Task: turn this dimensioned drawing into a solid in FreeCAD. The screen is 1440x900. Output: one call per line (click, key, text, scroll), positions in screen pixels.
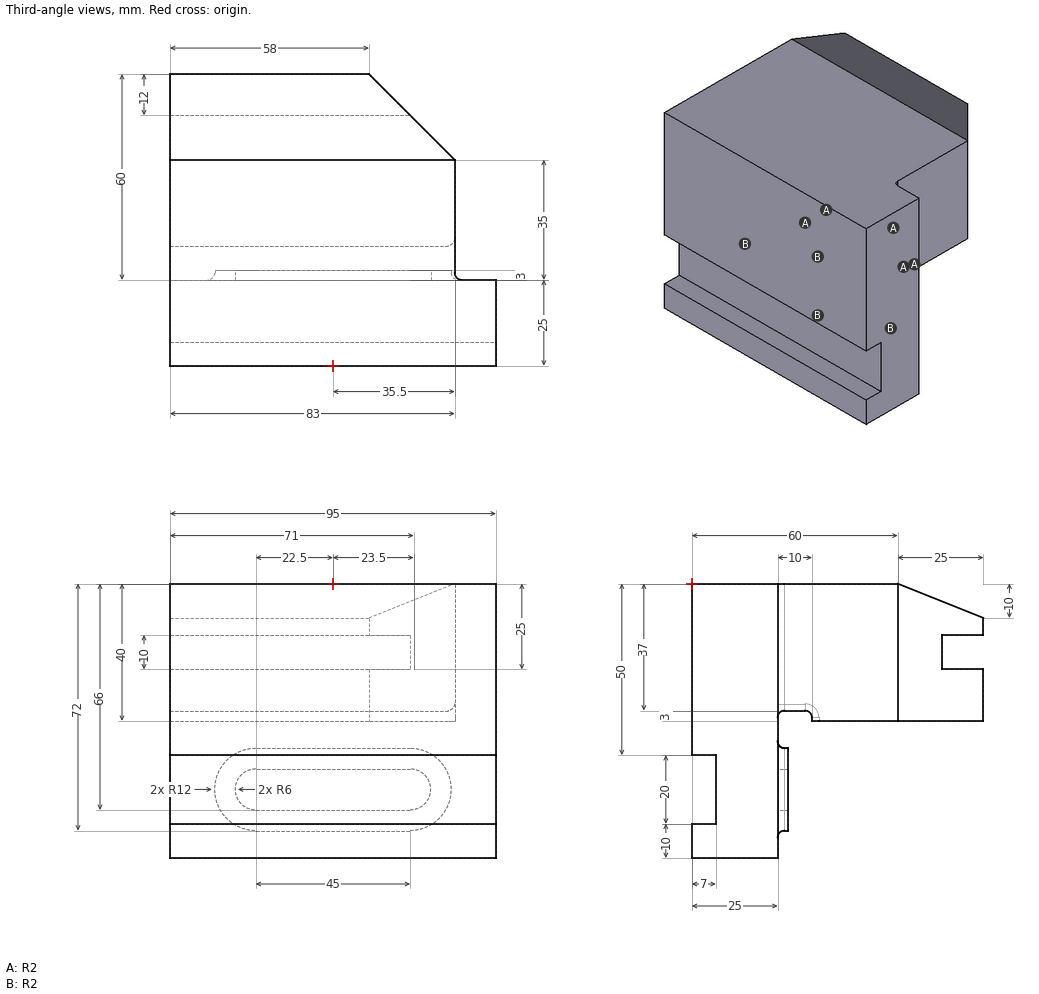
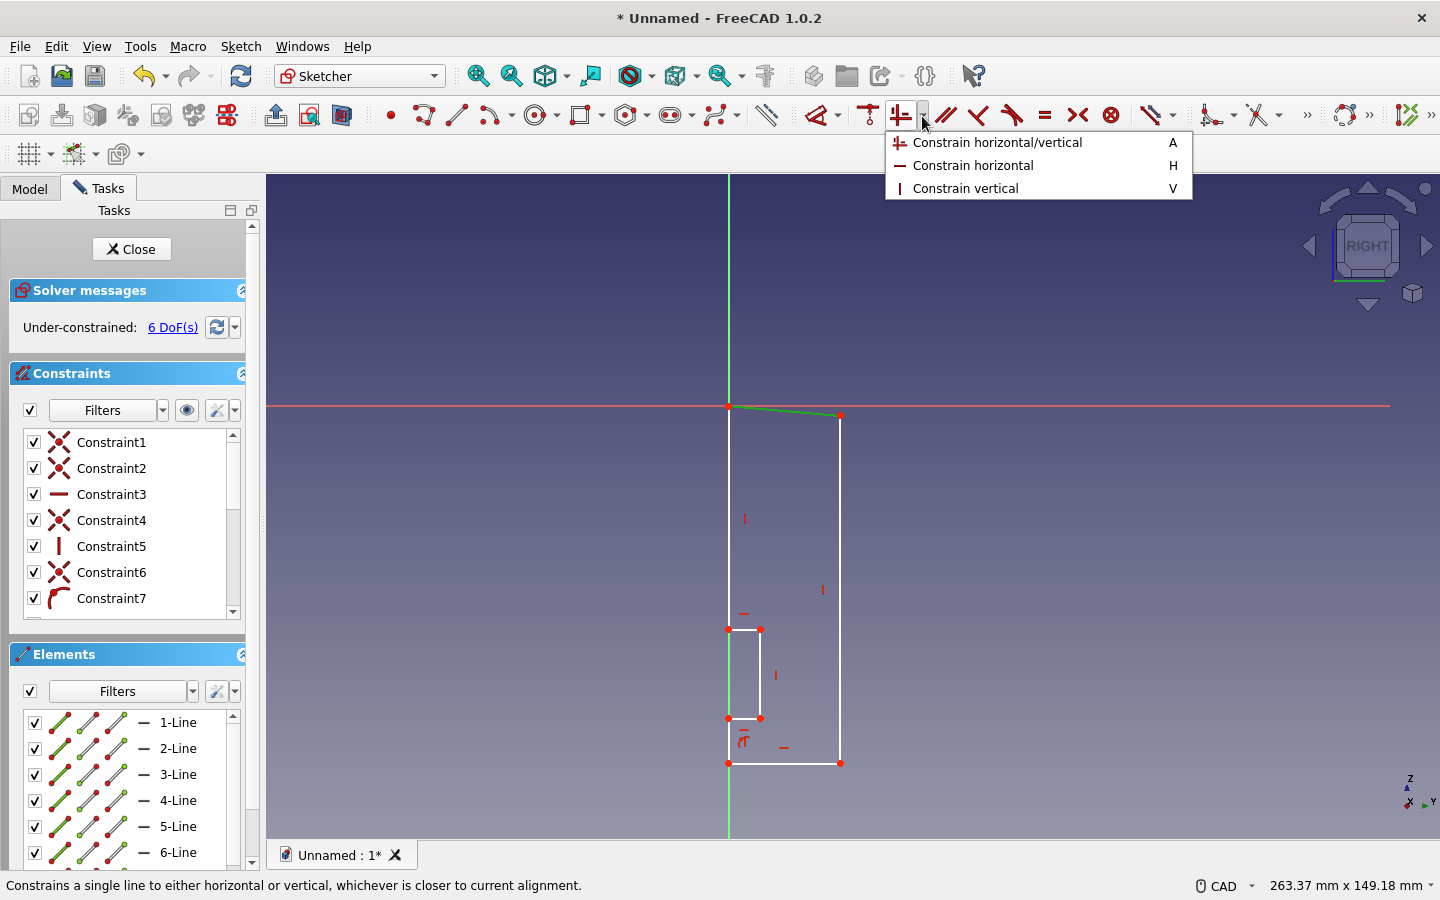
click(1039, 166)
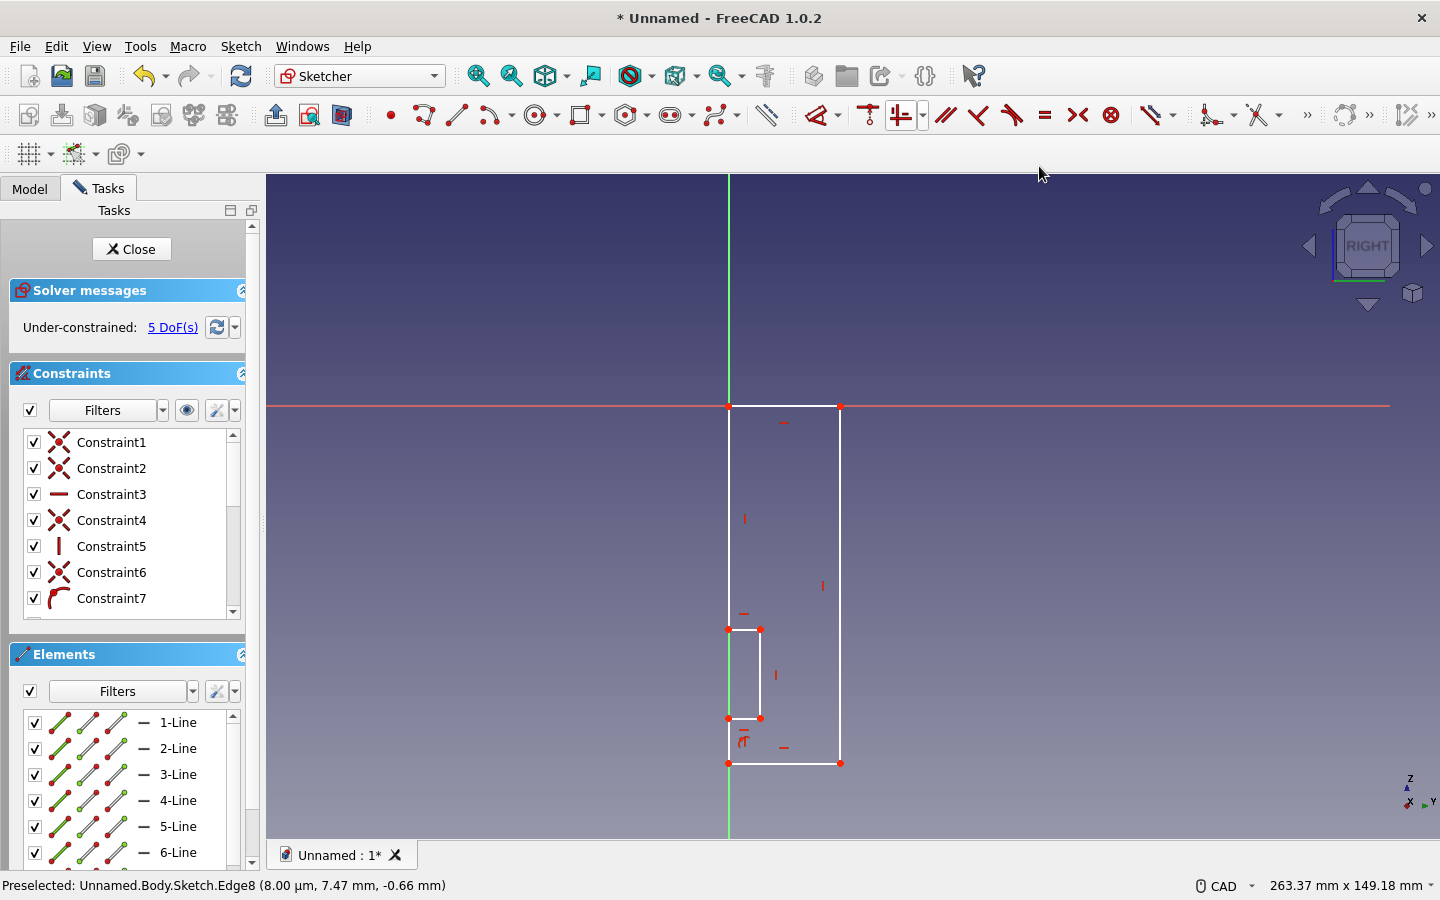
scroll(738, 630, up, 2)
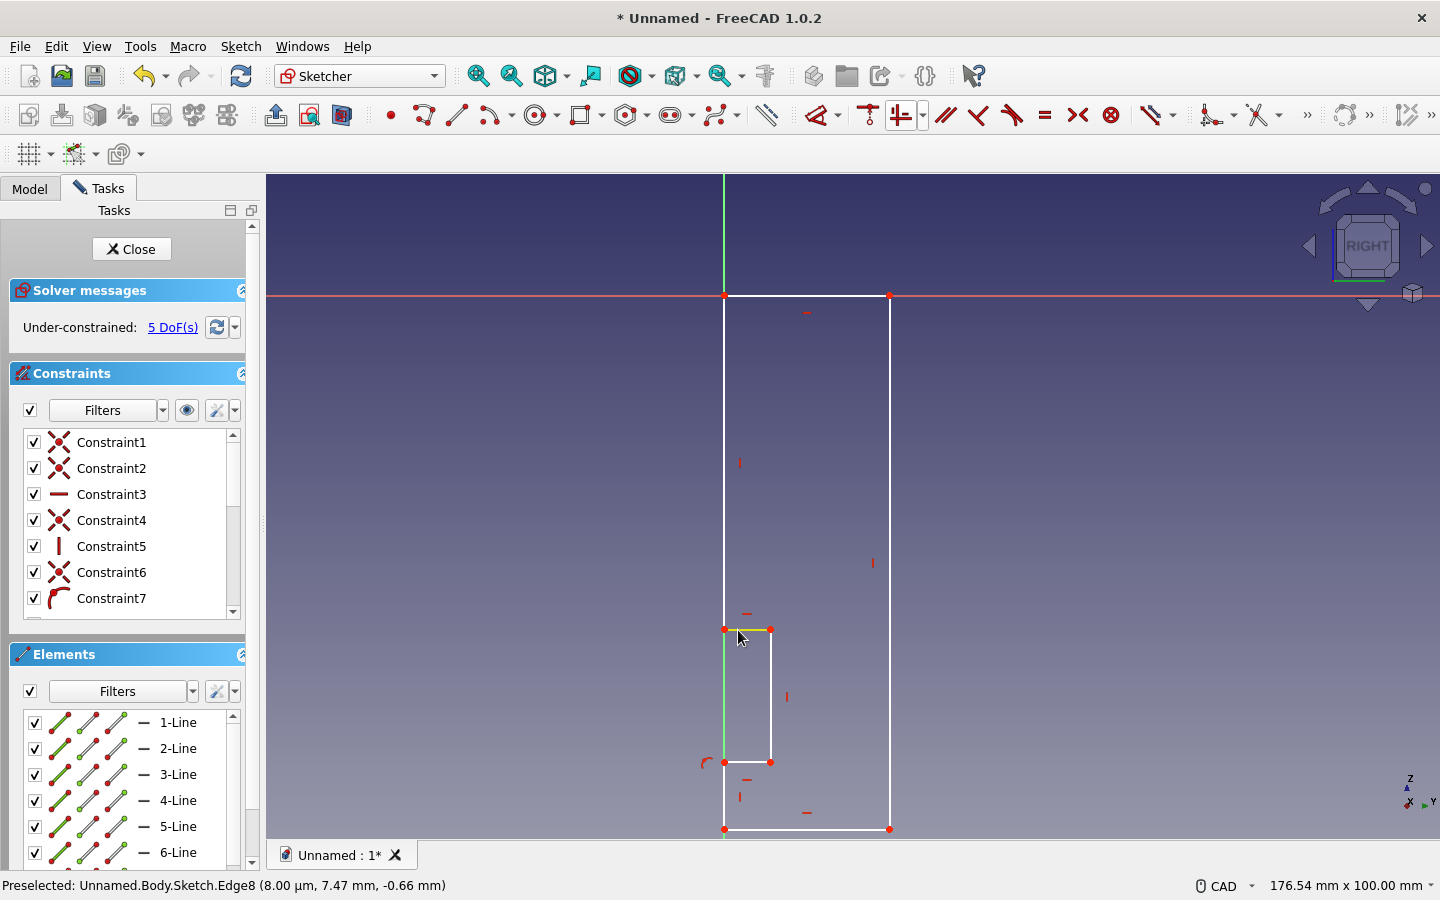
click(738, 630)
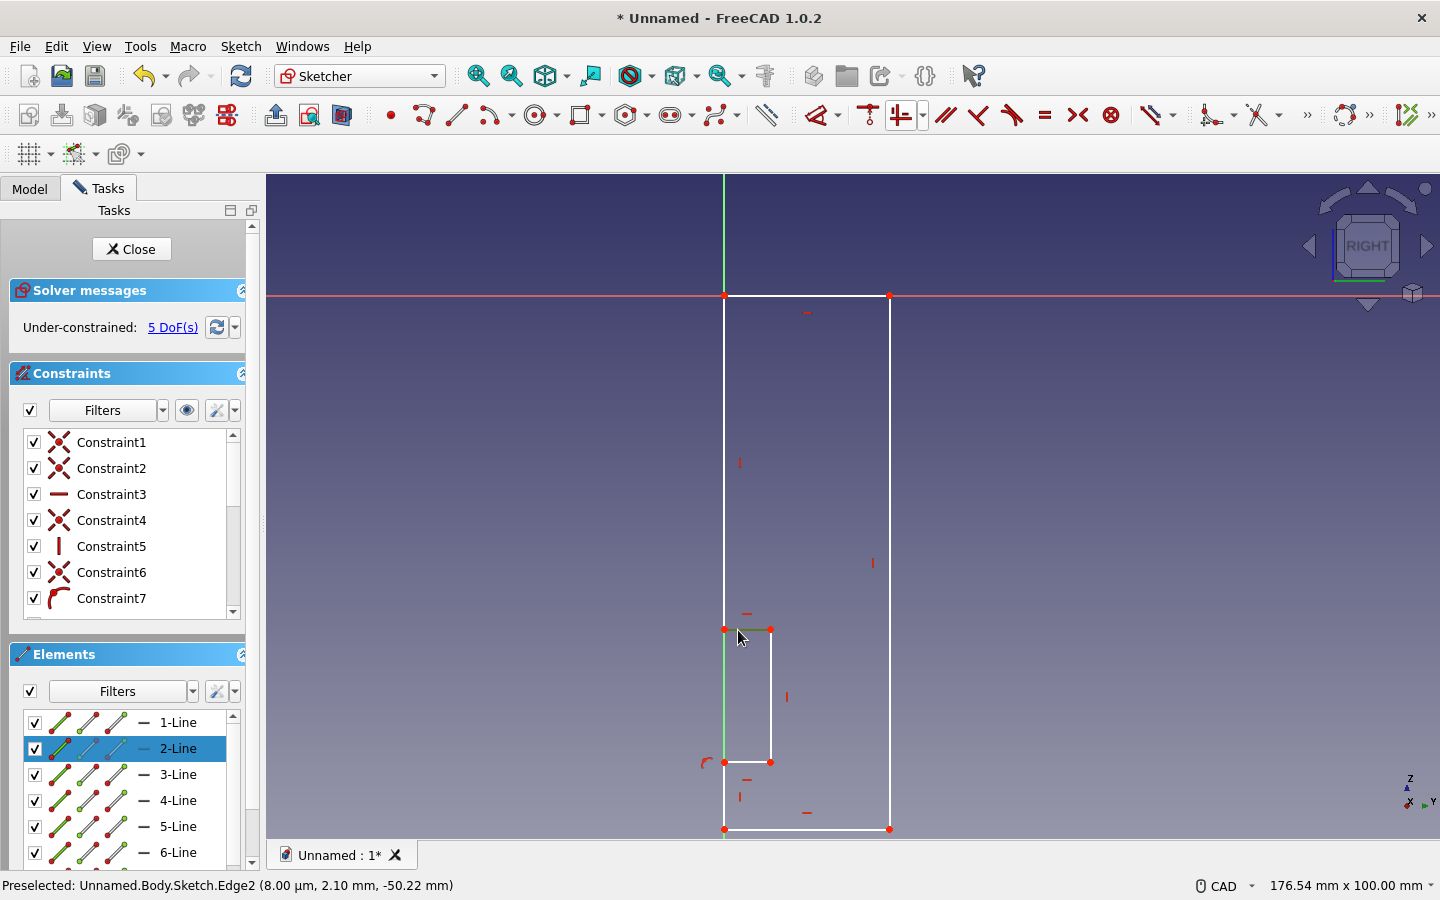
key(l)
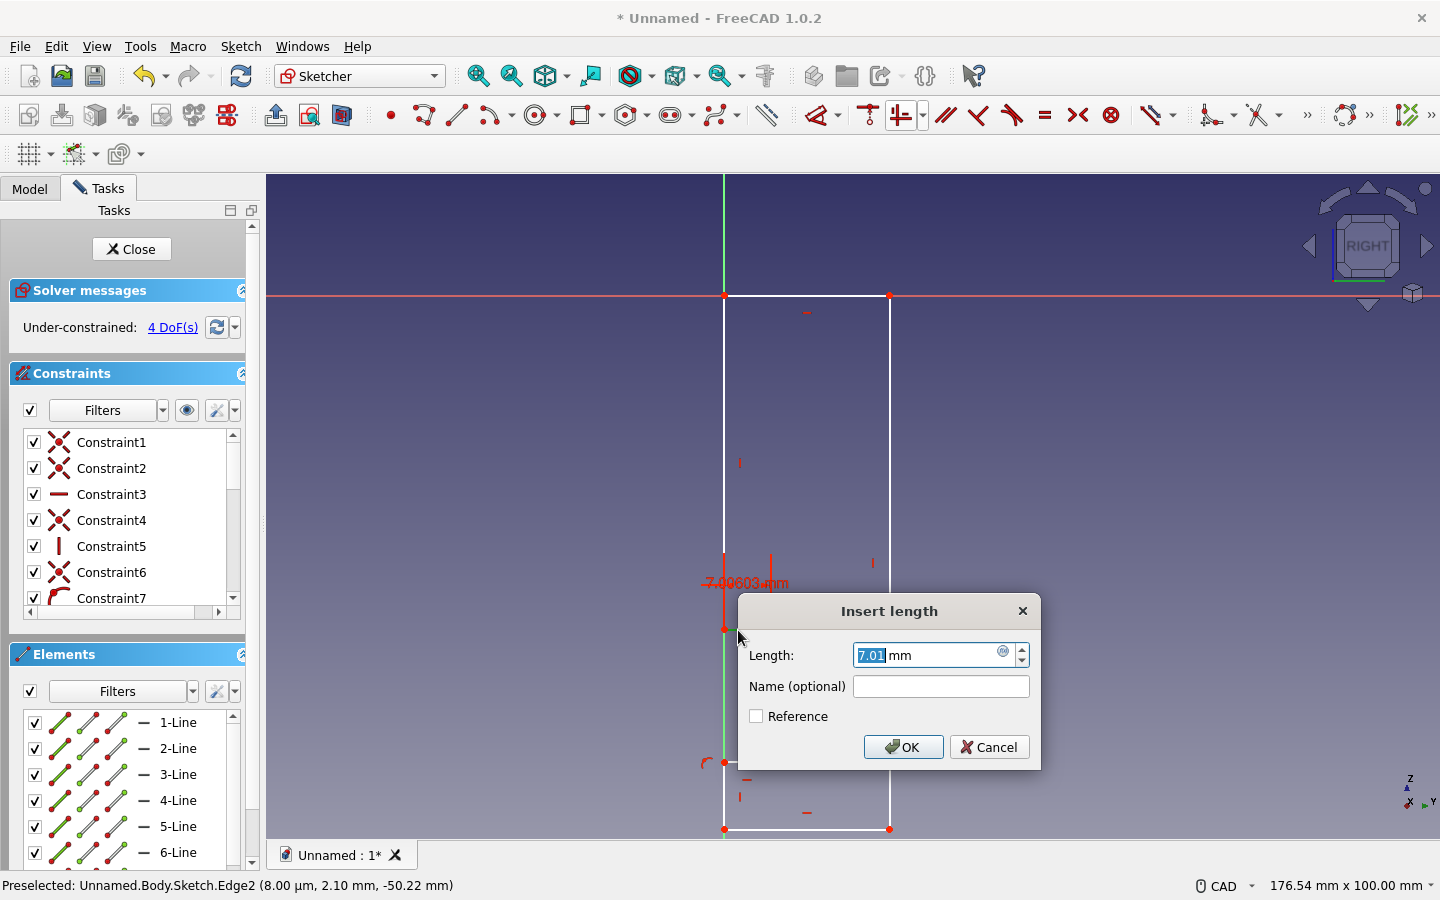
text(7)
key(Return)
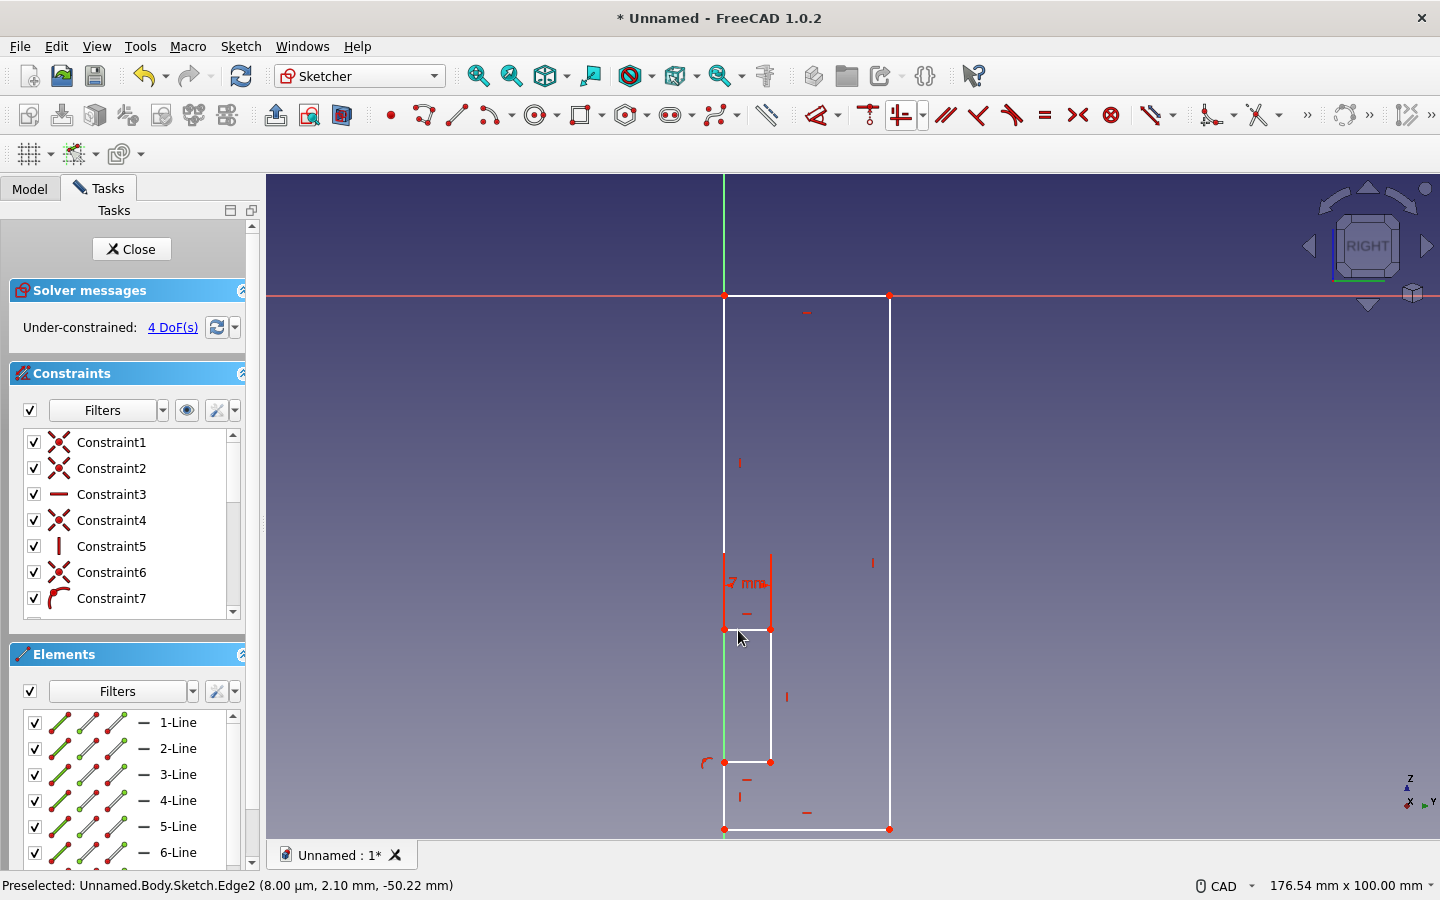
click(724, 396)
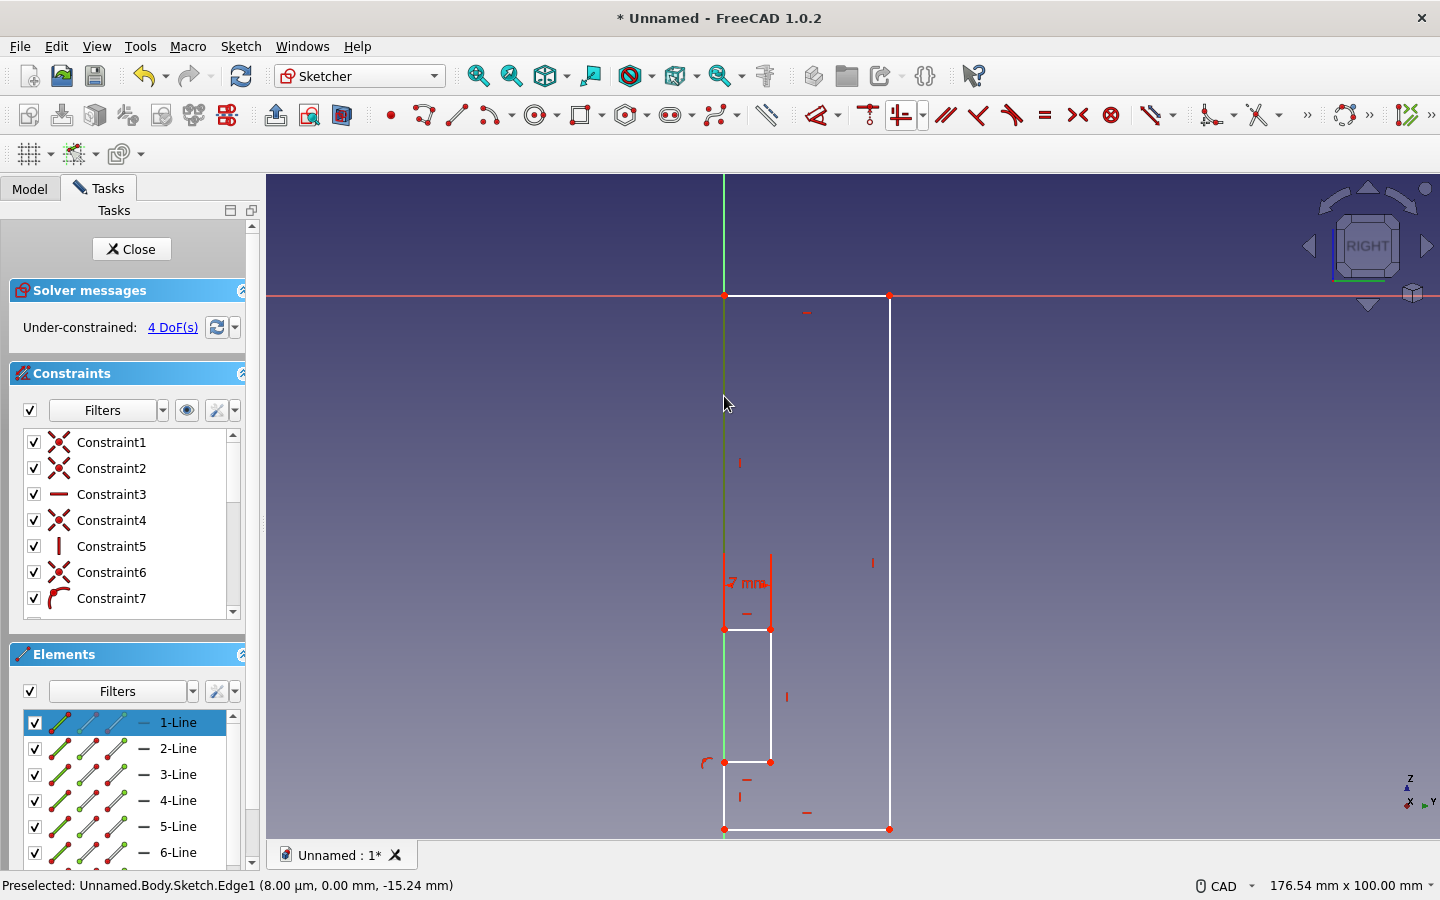
click(838, 116)